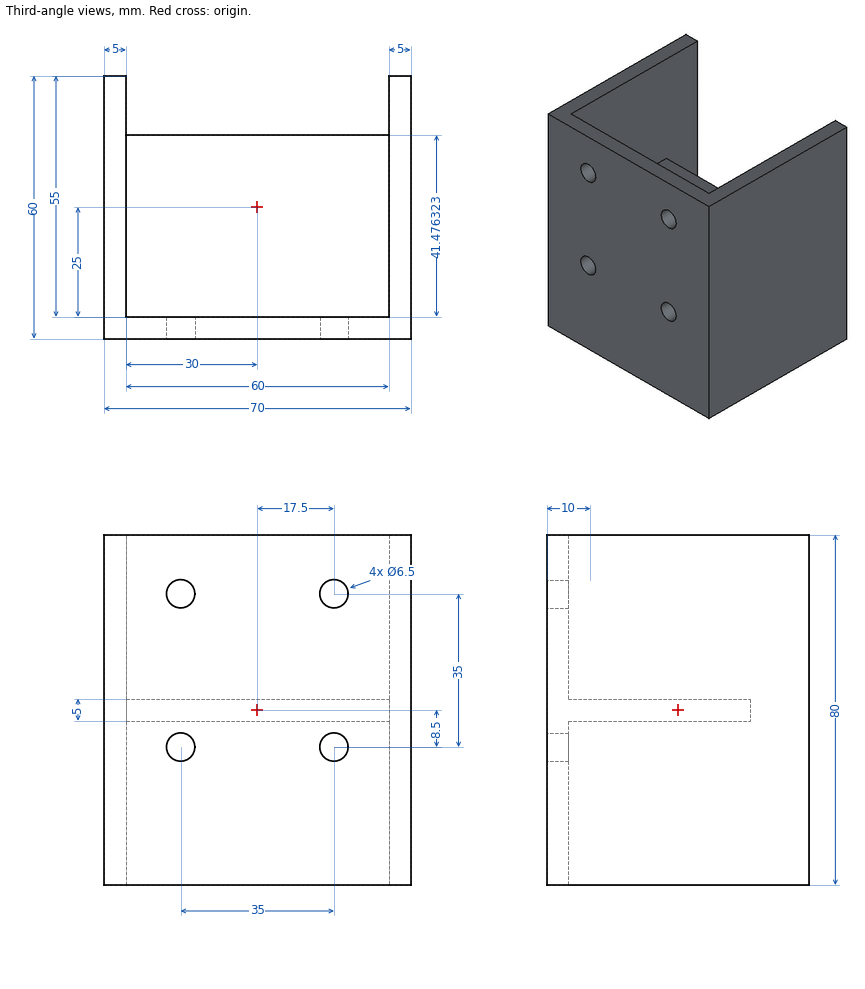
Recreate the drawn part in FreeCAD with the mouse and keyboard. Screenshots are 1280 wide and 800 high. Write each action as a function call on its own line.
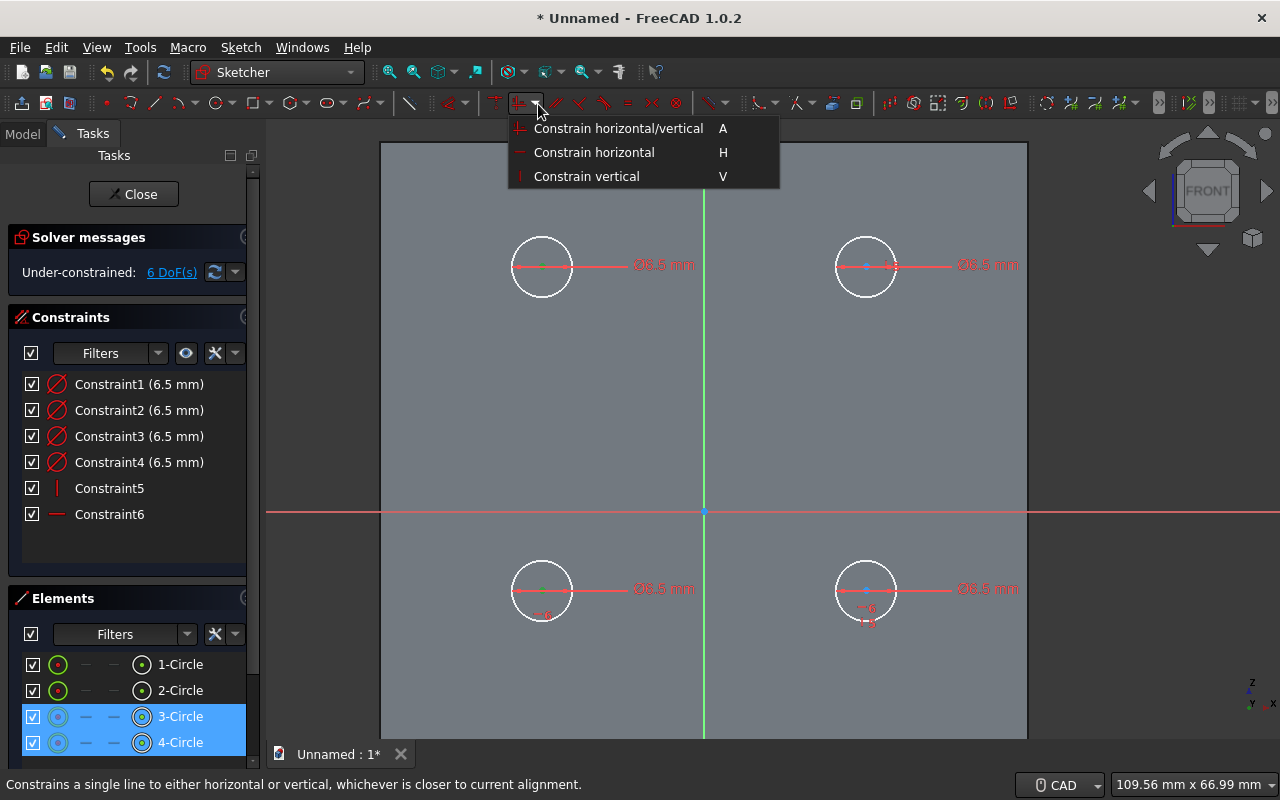
click(644, 176)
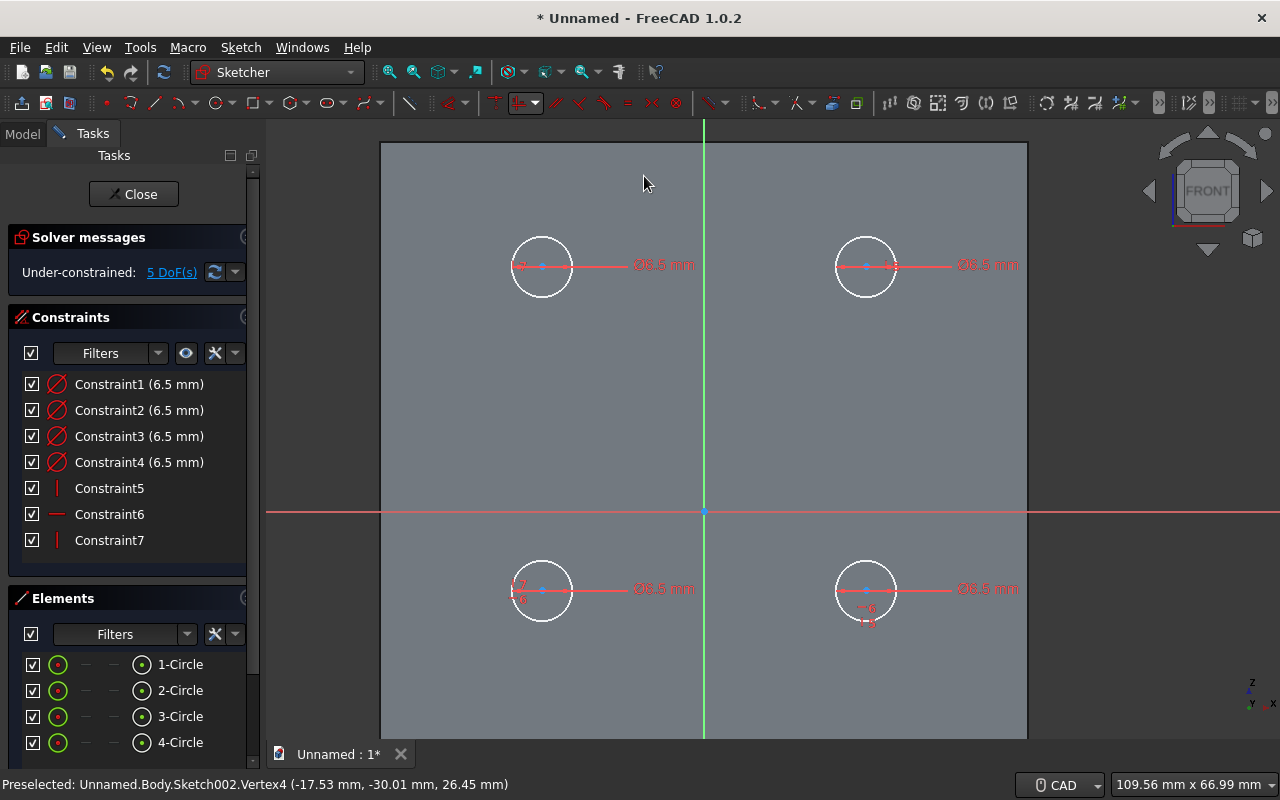
click(866, 267)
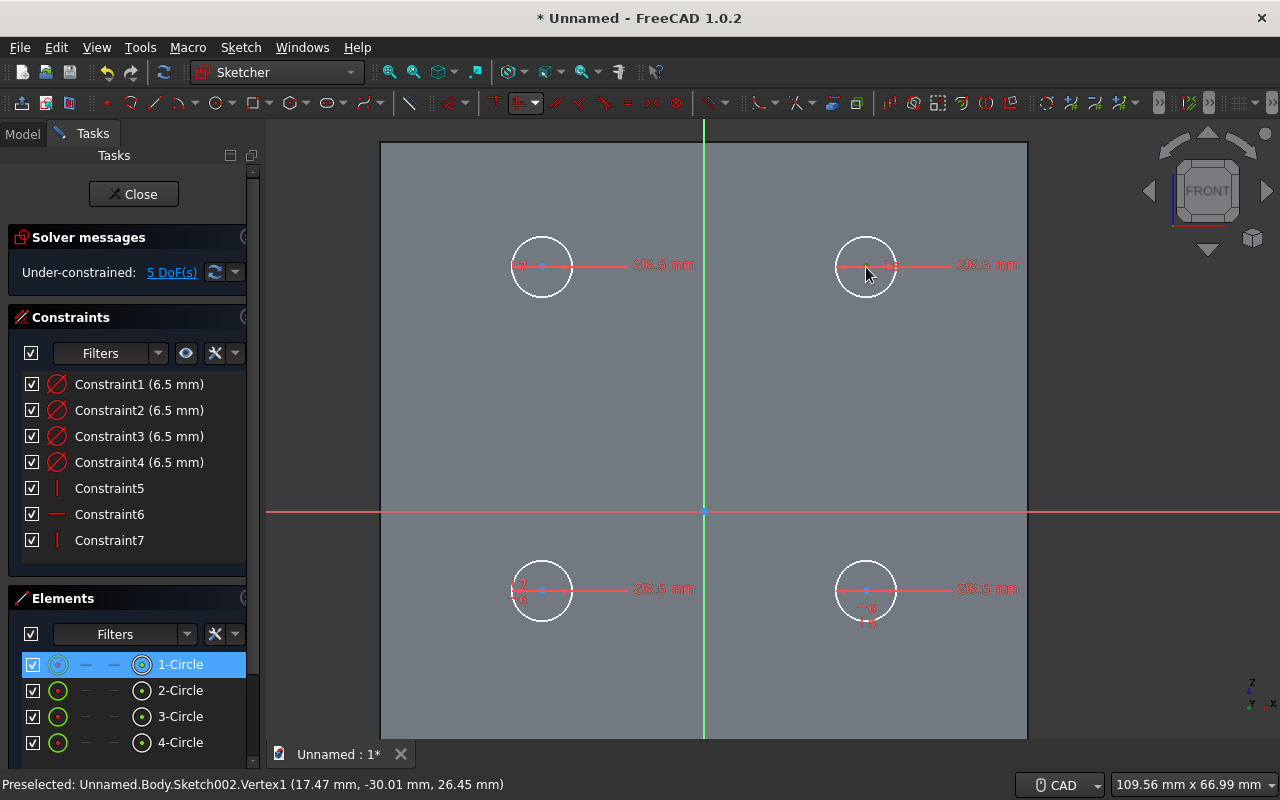
click(542, 267)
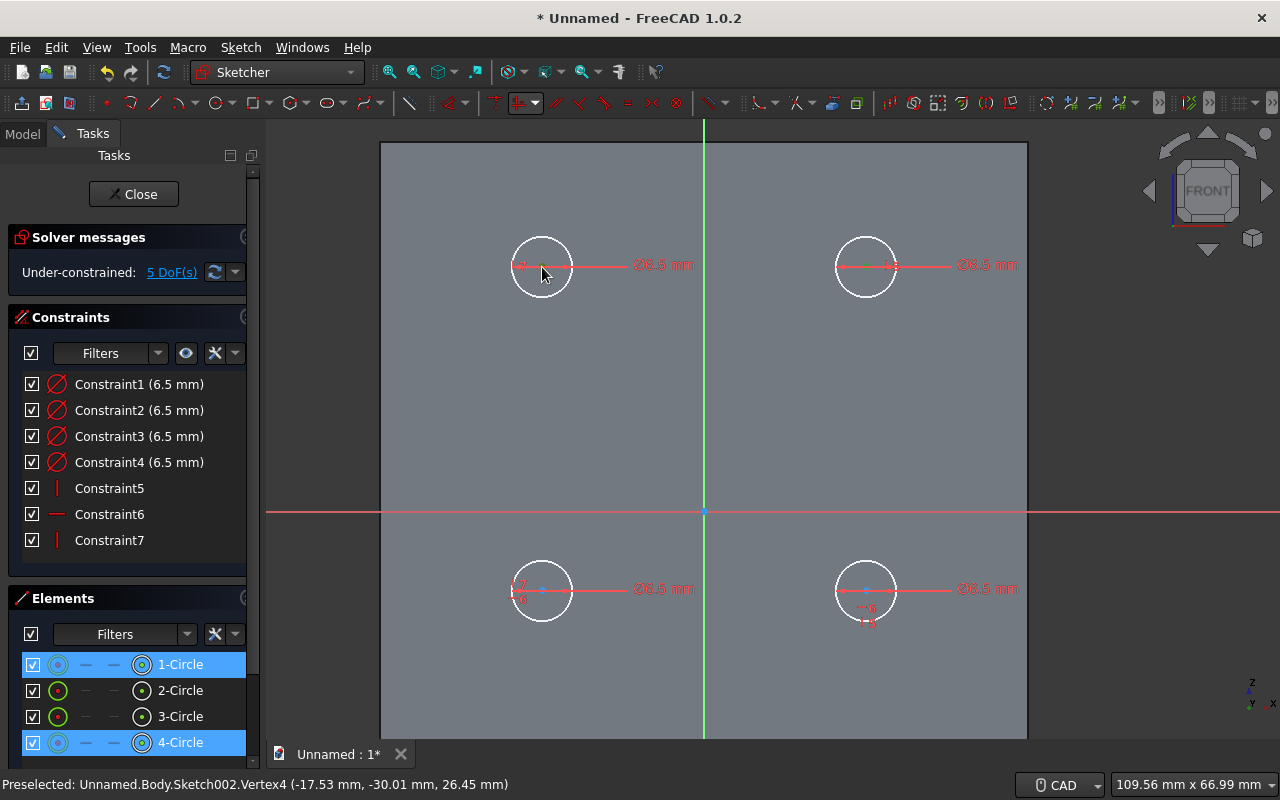
click(538, 104)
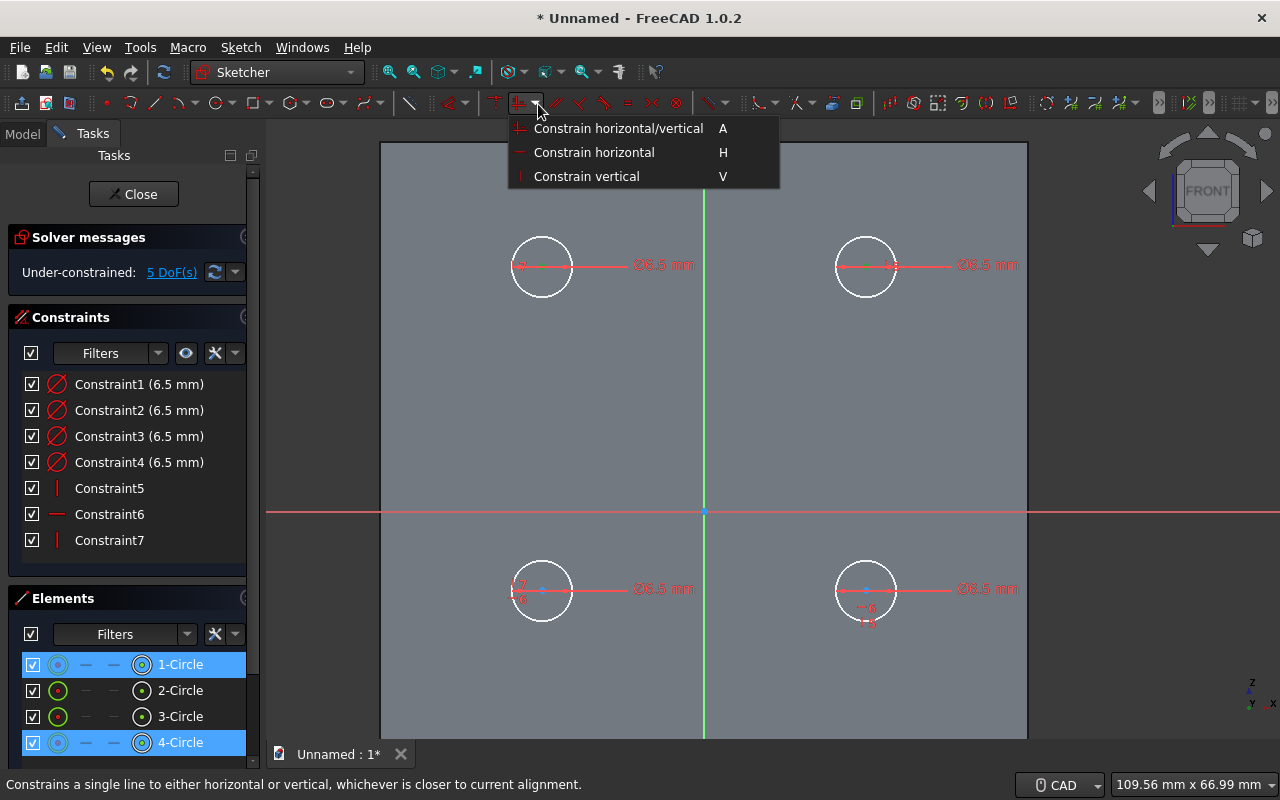
click(644, 152)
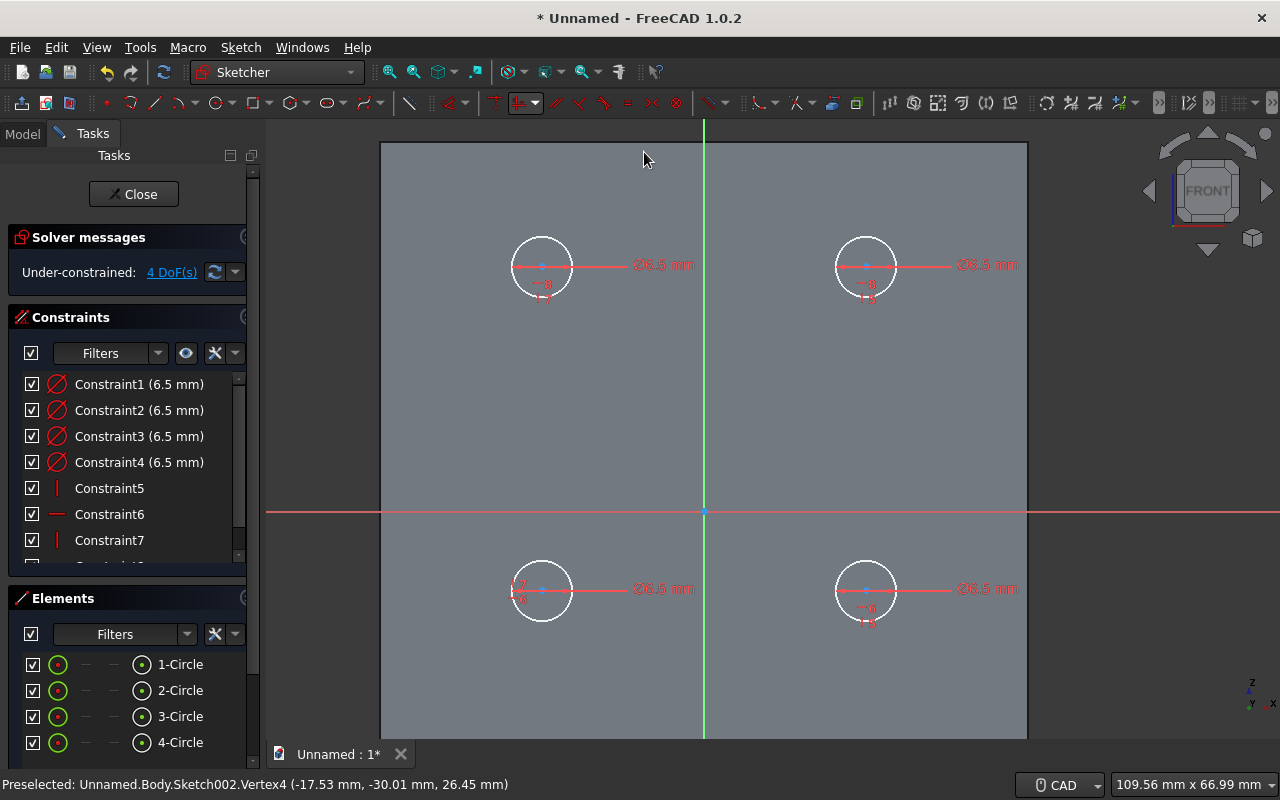
click(866, 591)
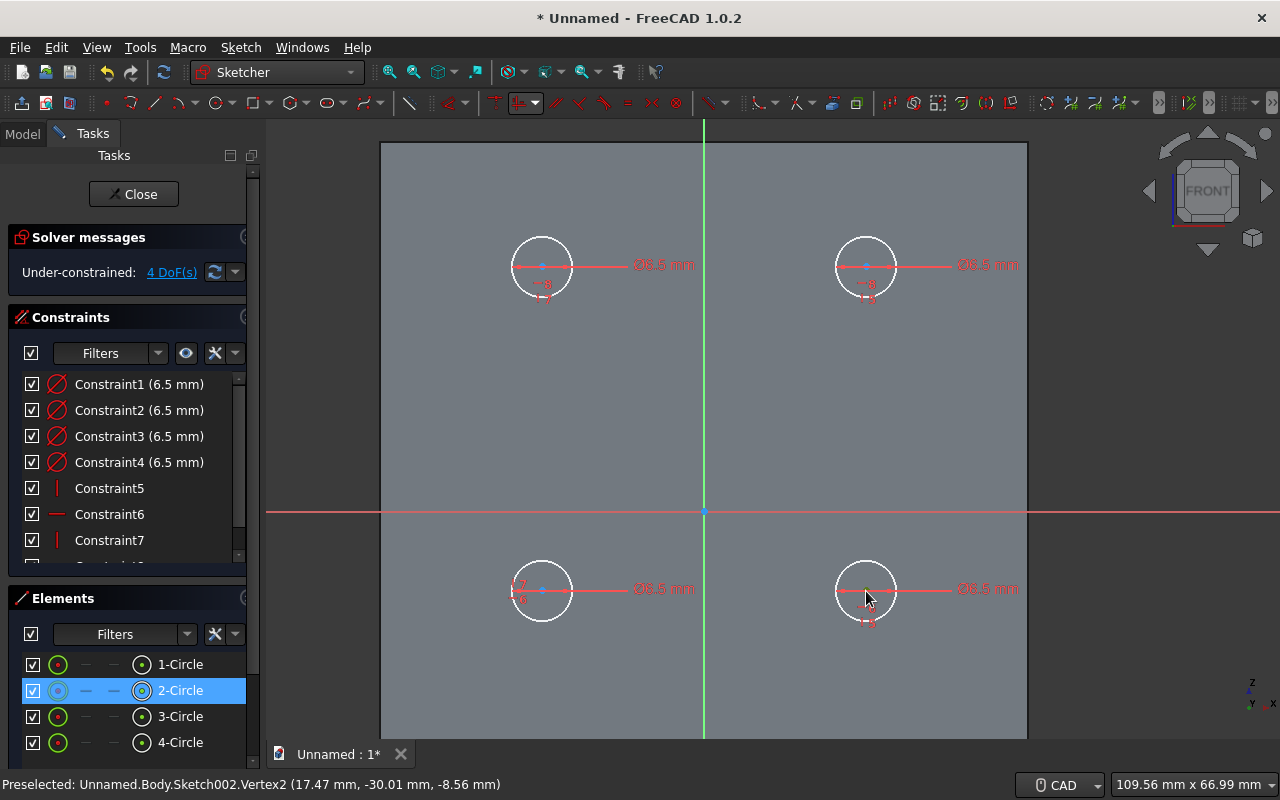
key(i)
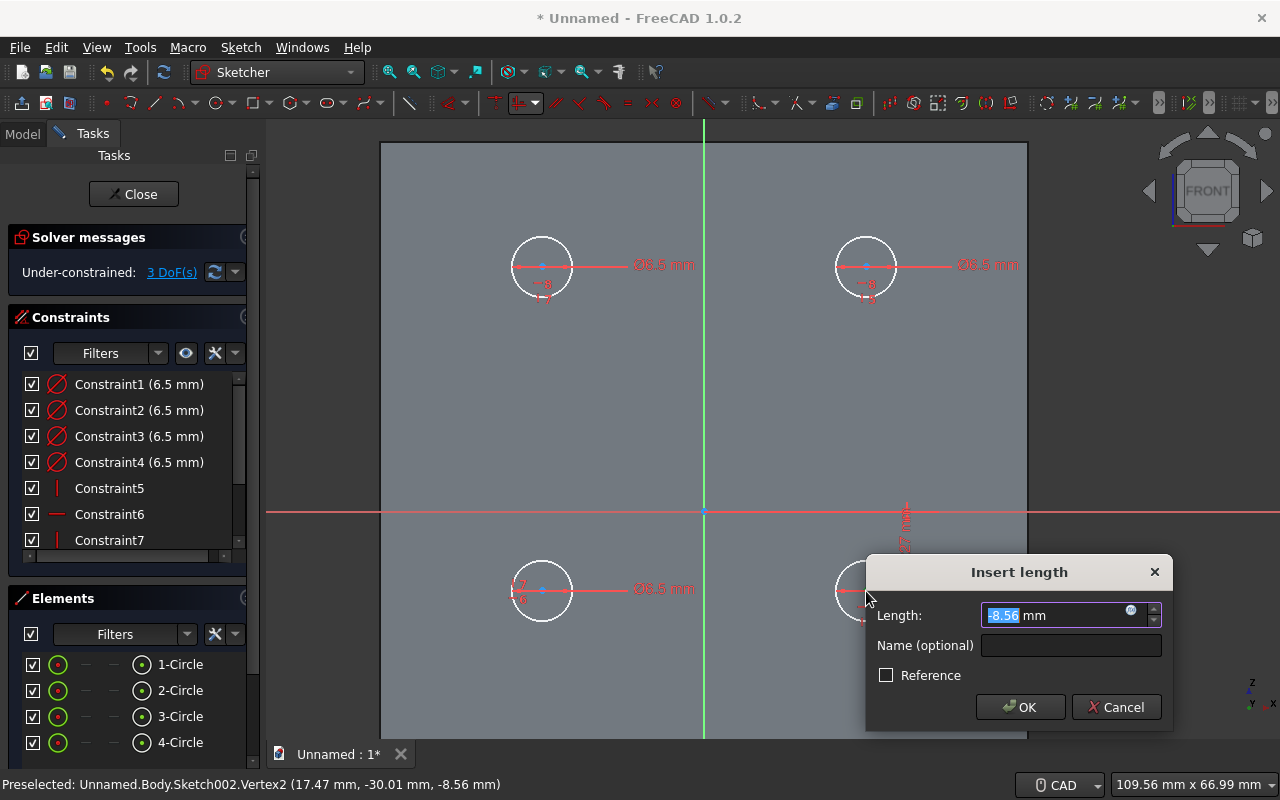
text(-8.5)
key(Return)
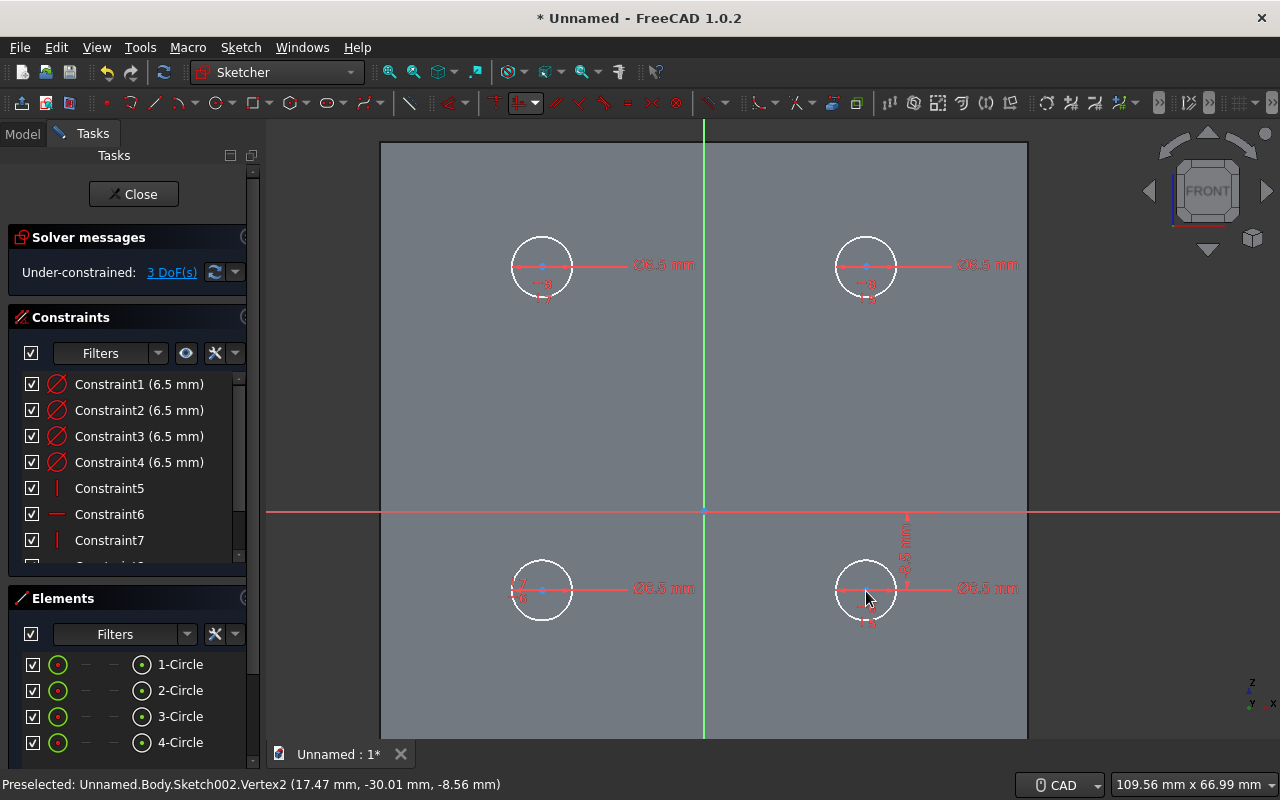
click(866, 267)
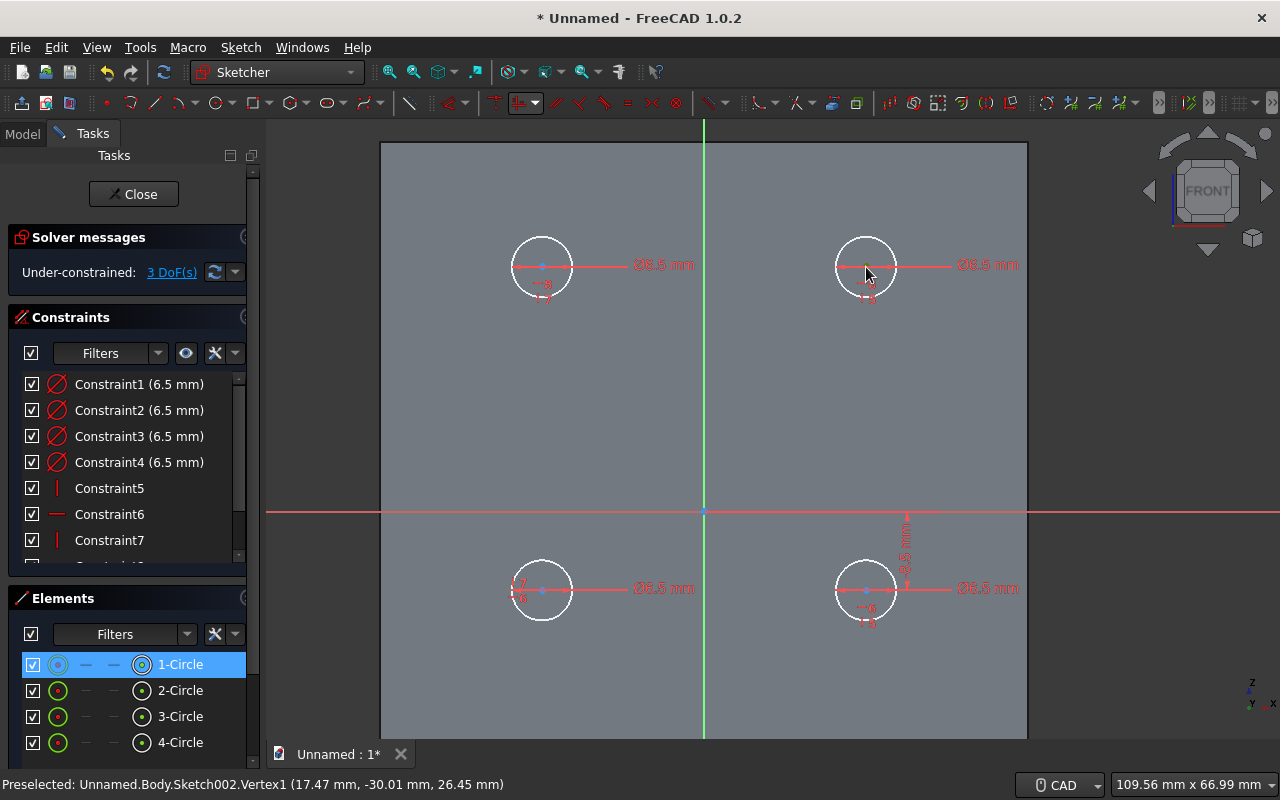
click(866, 590)